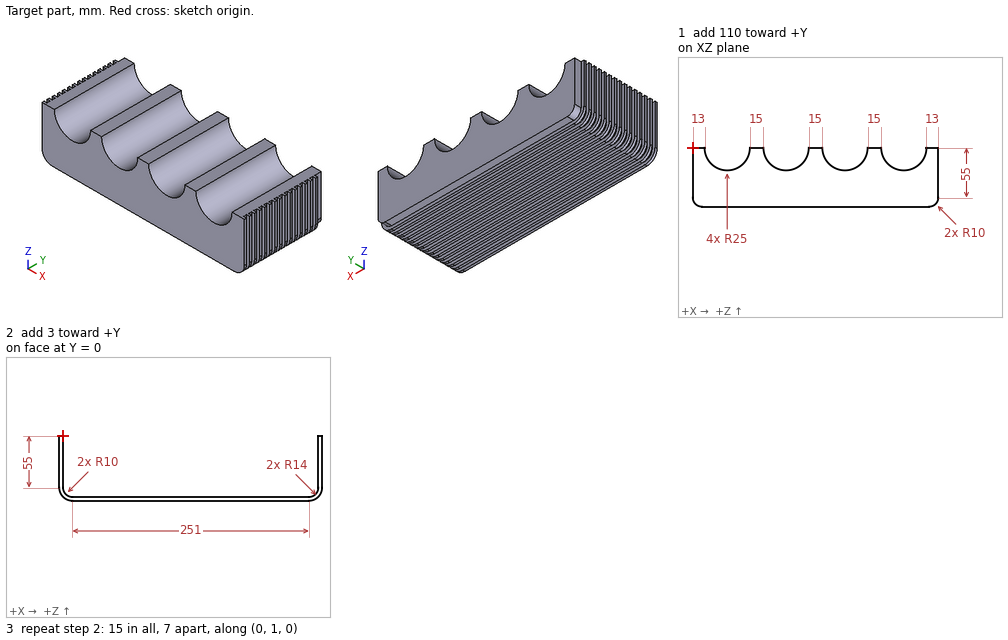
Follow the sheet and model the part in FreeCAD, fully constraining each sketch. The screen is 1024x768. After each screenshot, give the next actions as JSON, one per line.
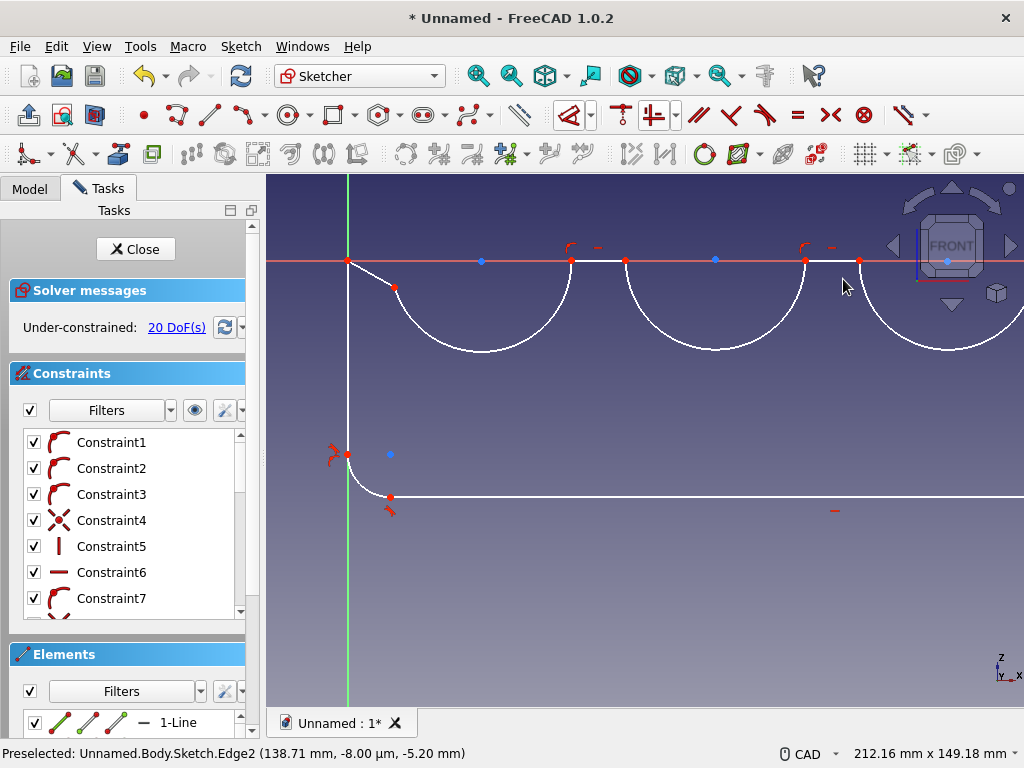
{"action": "scroll", "coordinate": [368, 492], "scroll_direction": "down", "scroll_amount": 4}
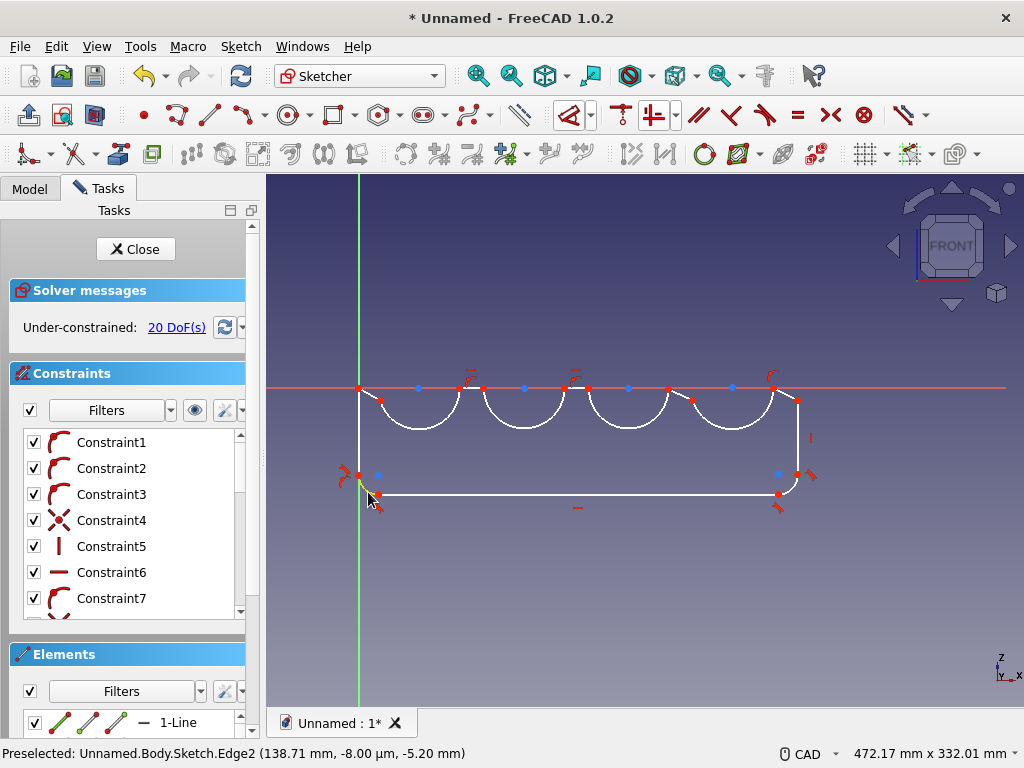
{"action": "scroll", "coordinate": [676, 393], "scroll_direction": "up", "scroll_amount": 6}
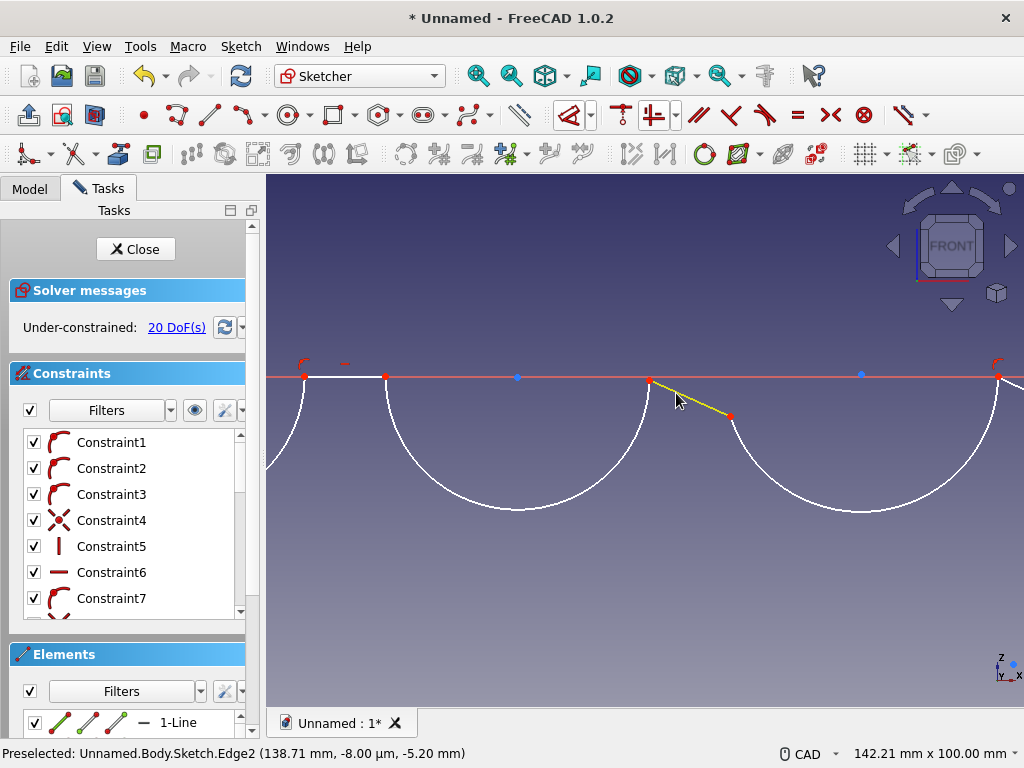
{"action": "left_click", "coordinate": [674, 391]}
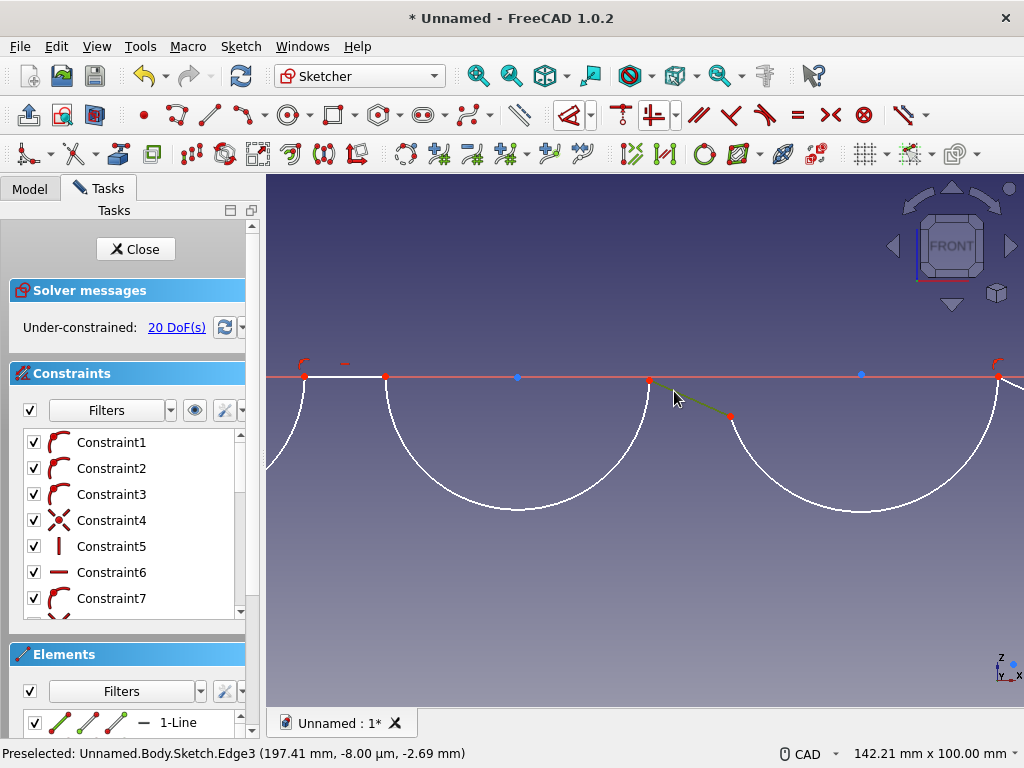
{"action": "key", "text": "h"}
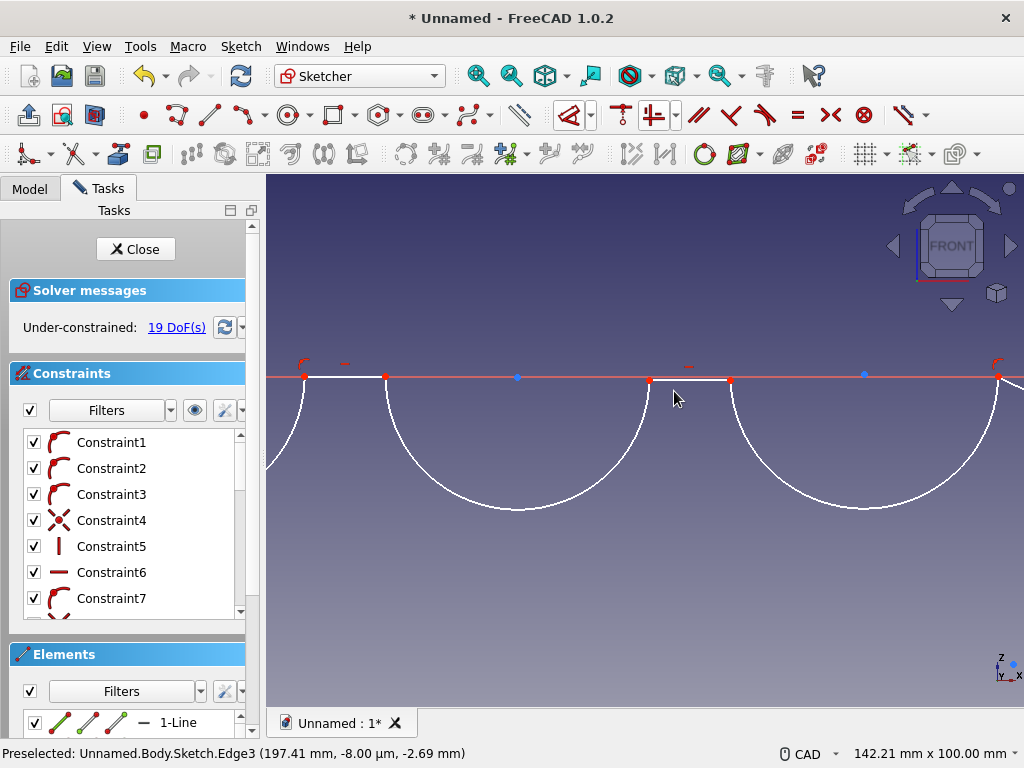
{"action": "scroll", "coordinate": [677, 393], "scroll_direction": "down", "scroll_amount": 6}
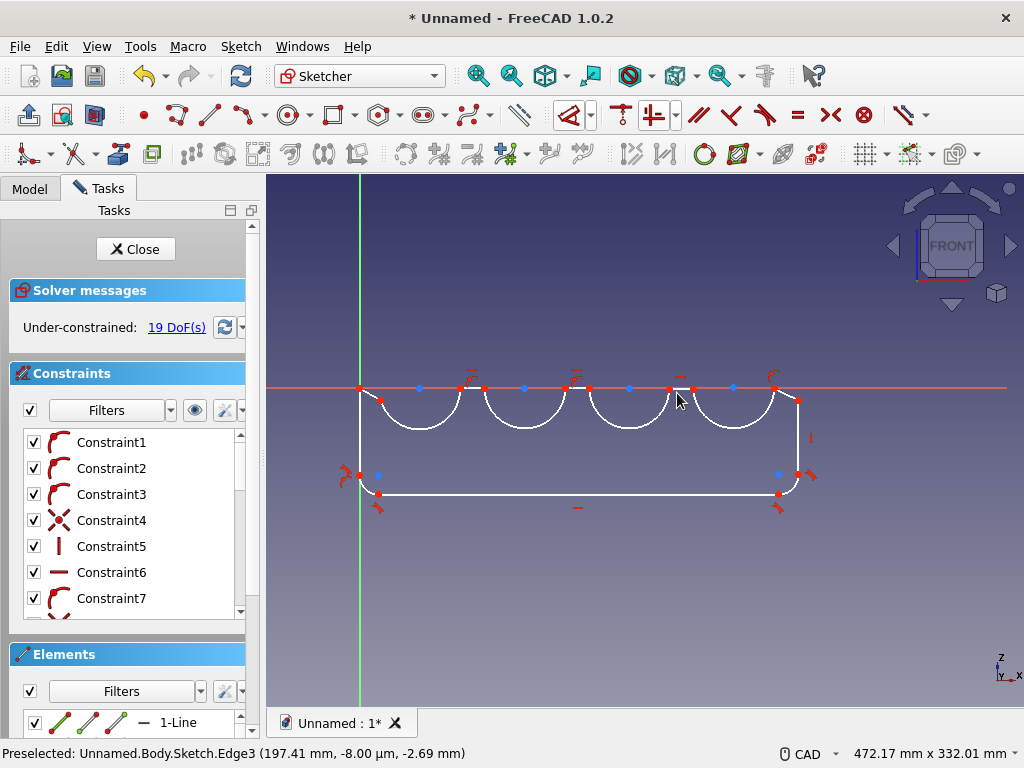
{"action": "scroll", "coordinate": [781, 392], "scroll_direction": "up", "scroll_amount": 7}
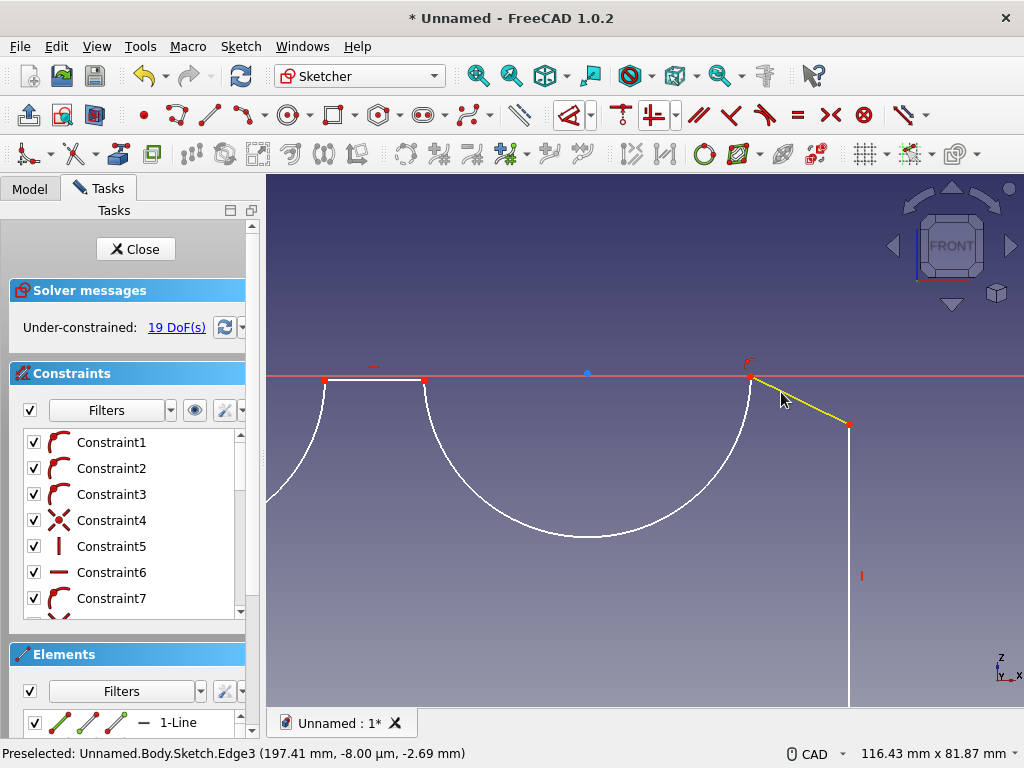
{"action": "left_click", "coordinate": [780, 391]}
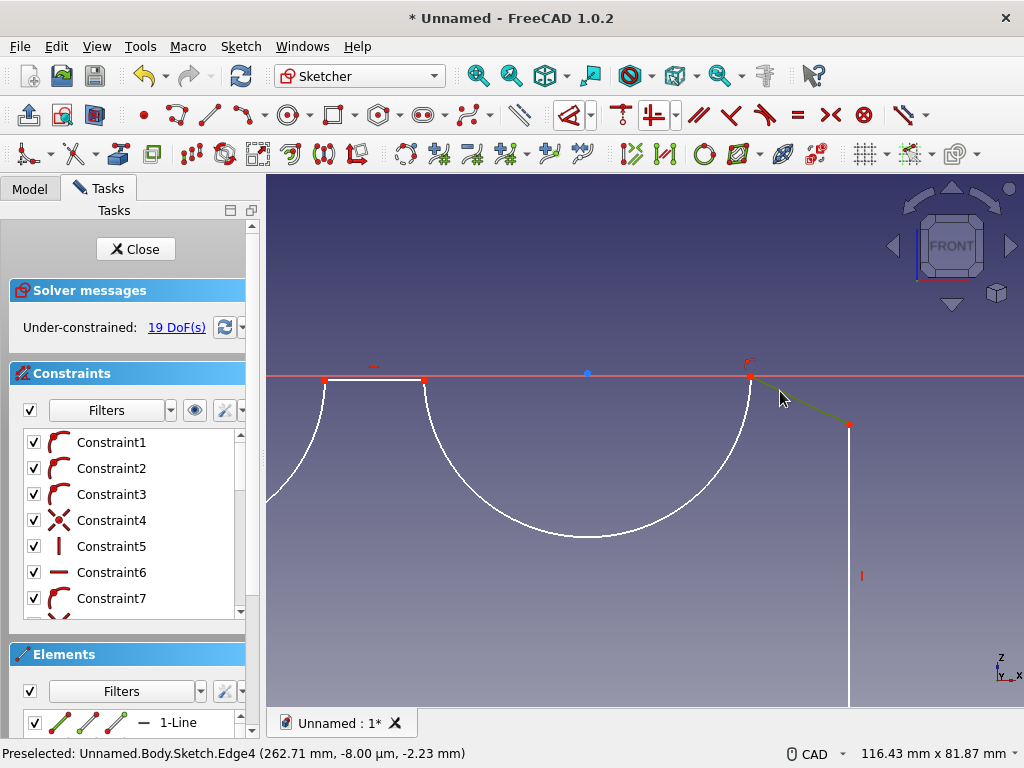
{"action": "left_click", "coordinate": [676, 116]}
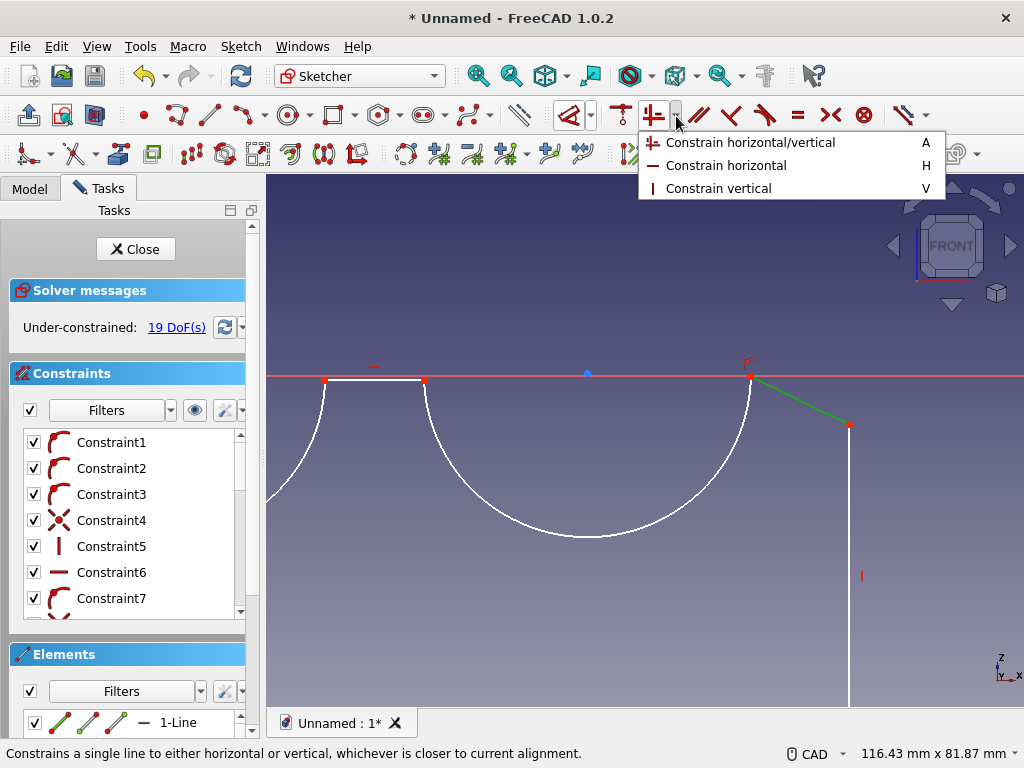
{"action": "left_click", "coordinate": [792, 166]}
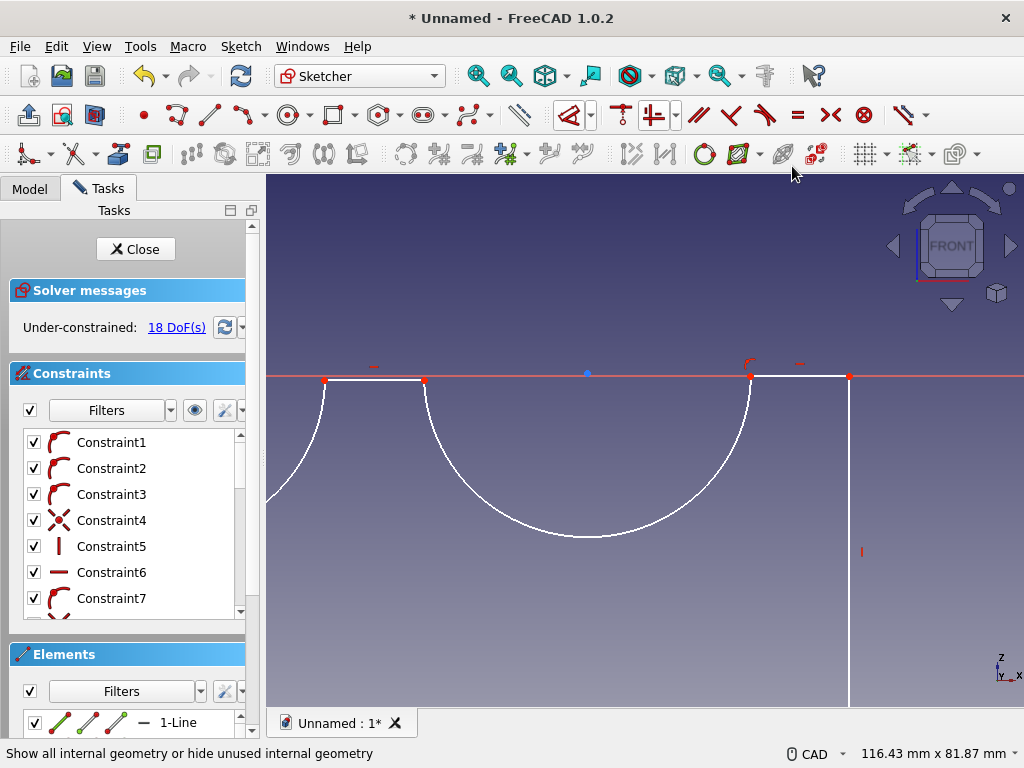
{"action": "scroll", "coordinate": [781, 392], "scroll_direction": "down", "scroll_amount": 7}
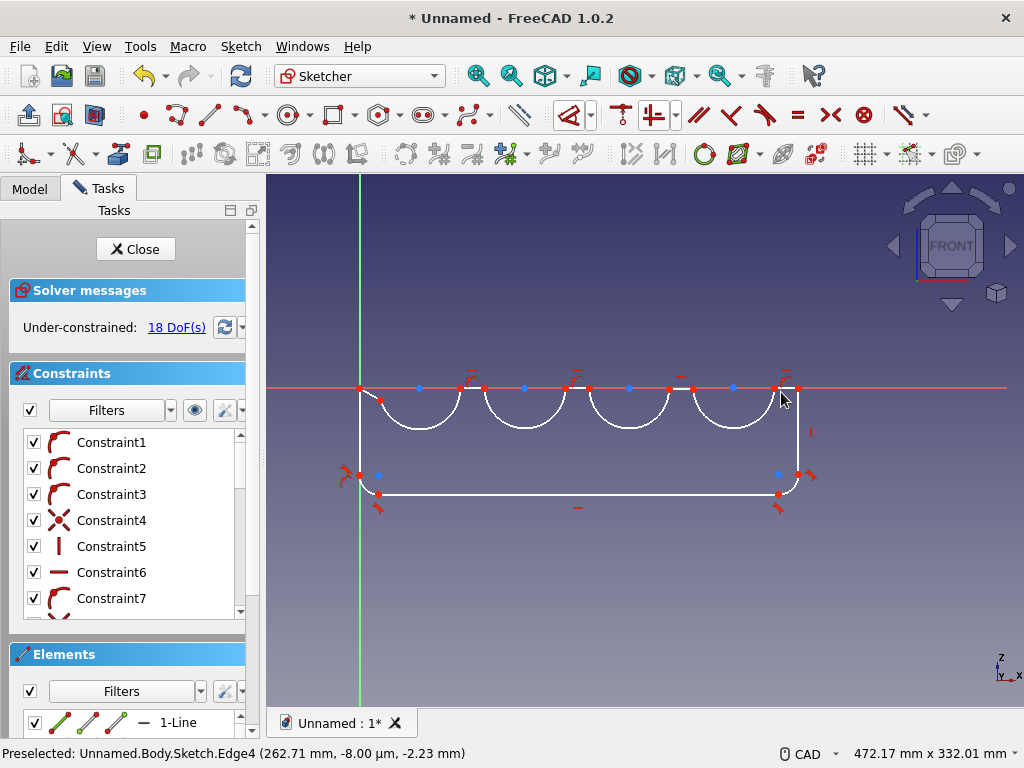
{"action": "scroll", "coordinate": [366, 392], "scroll_direction": "up", "scroll_amount": 7}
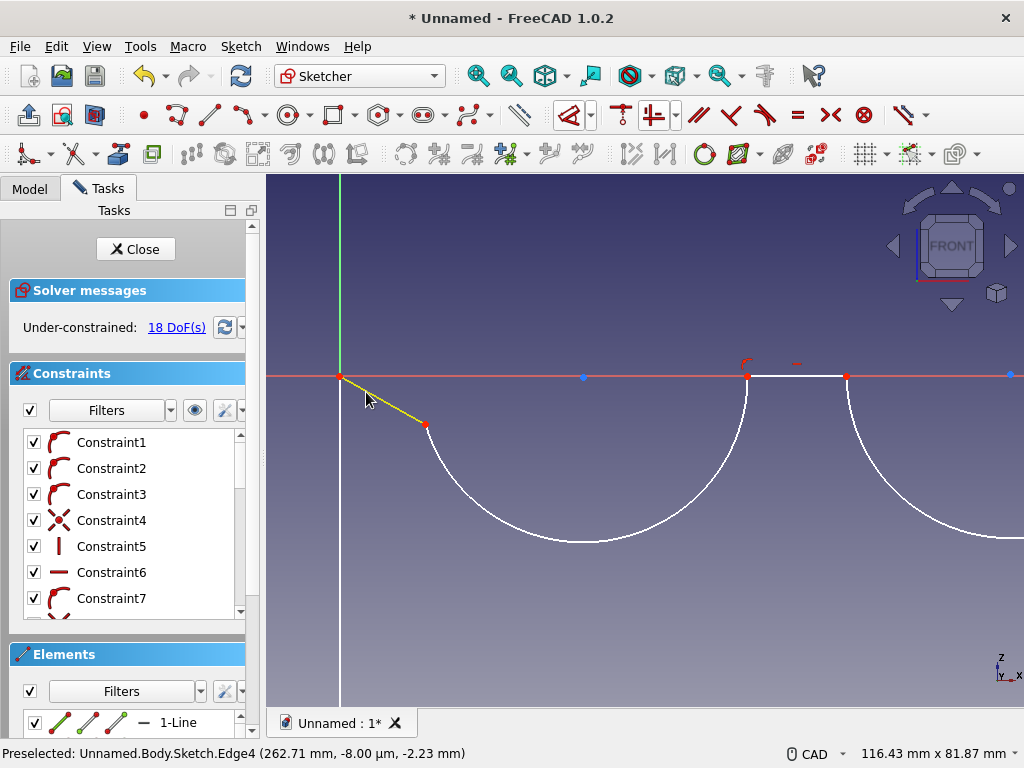
{"action": "left_click", "coordinate": [366, 391]}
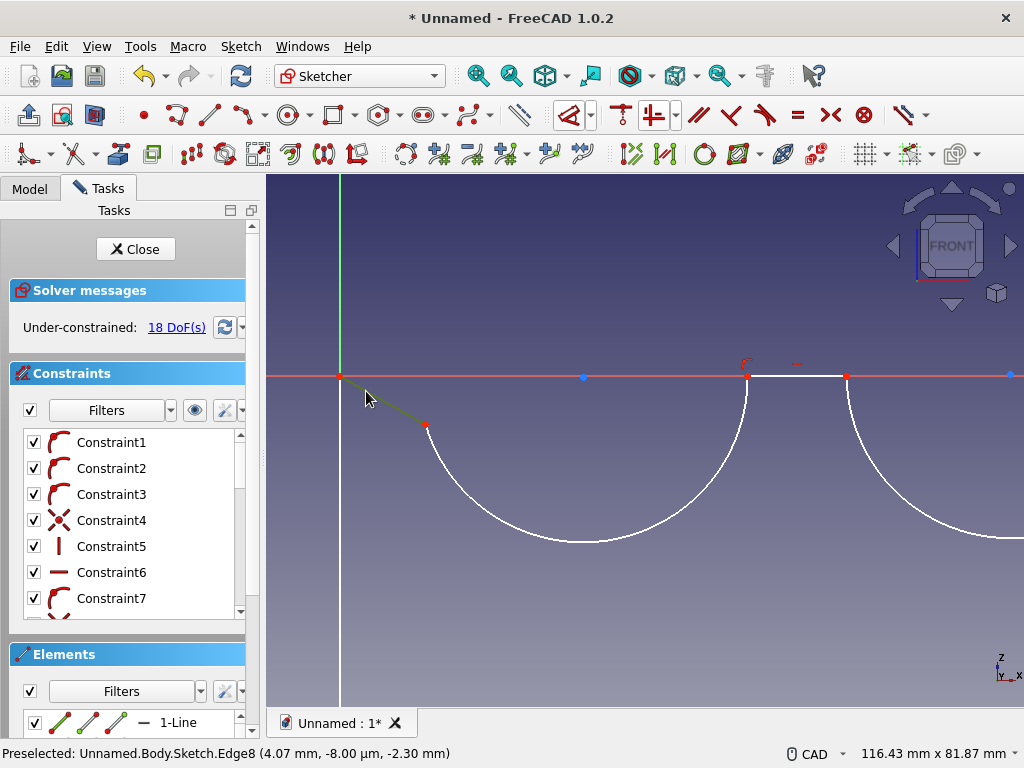
{"action": "key", "text": "h"}